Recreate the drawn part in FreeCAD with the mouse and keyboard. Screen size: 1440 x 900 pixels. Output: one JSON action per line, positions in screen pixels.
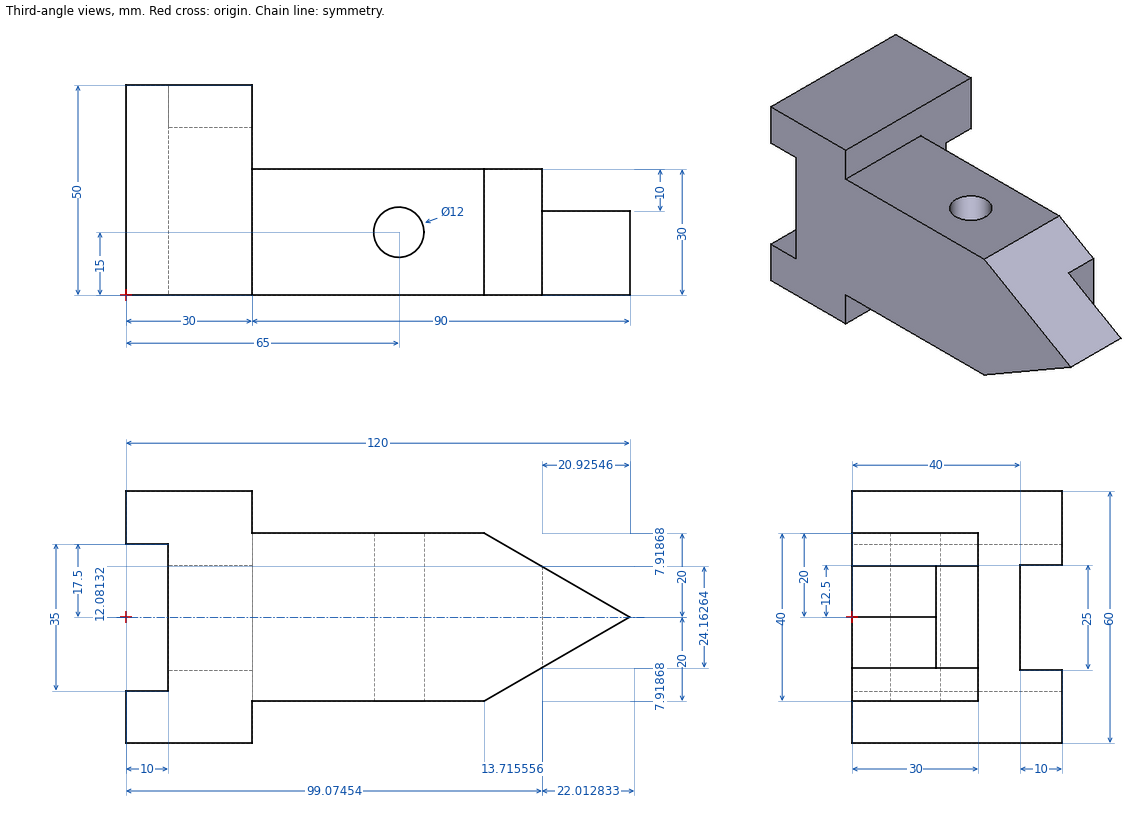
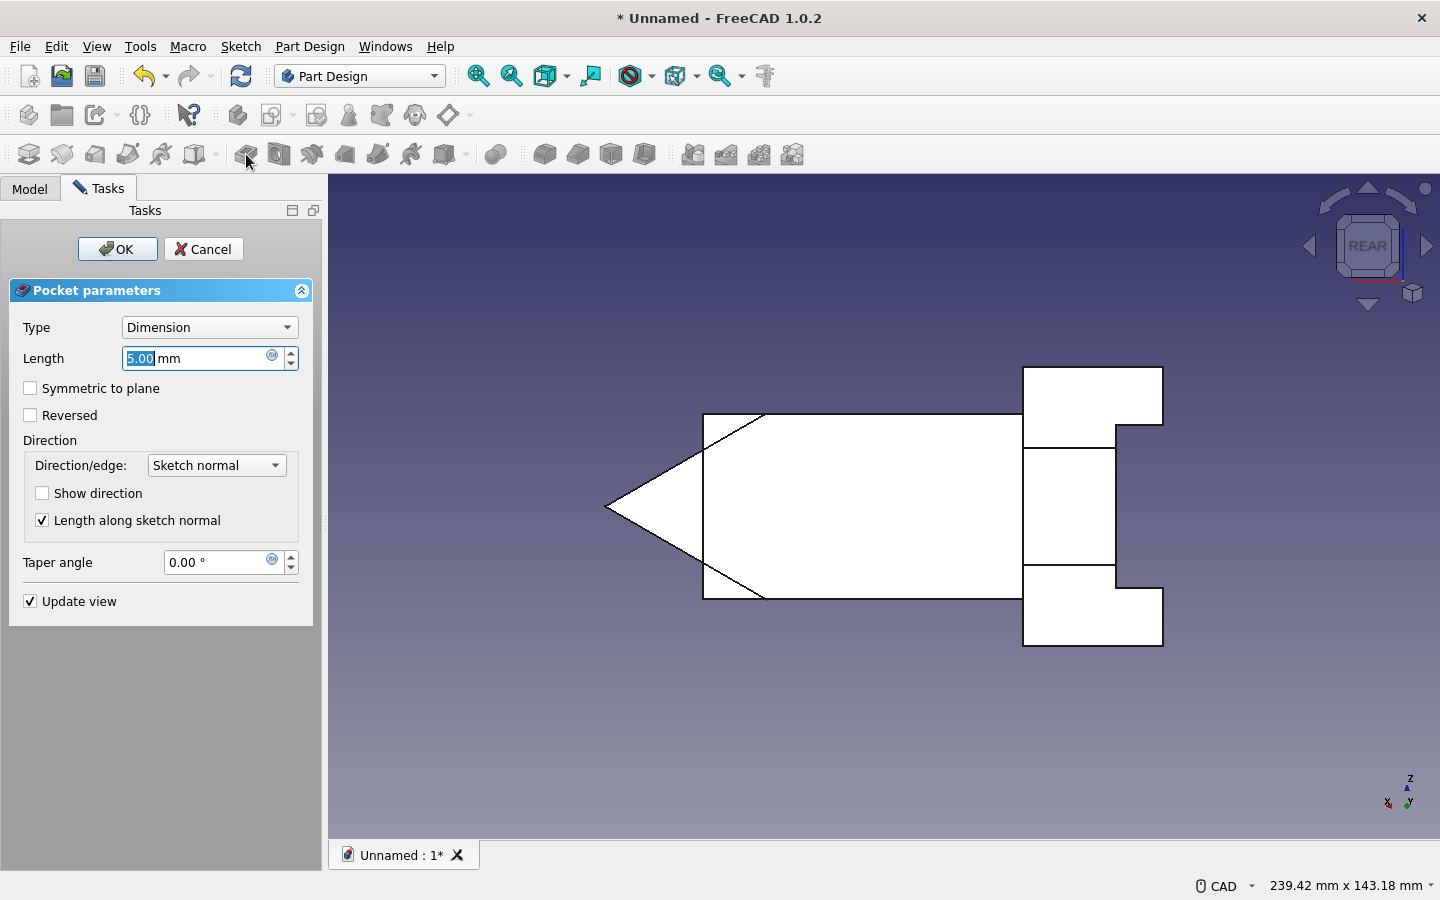
{"action": "type", "text": "30"}
{"action": "key", "text": "Tab"}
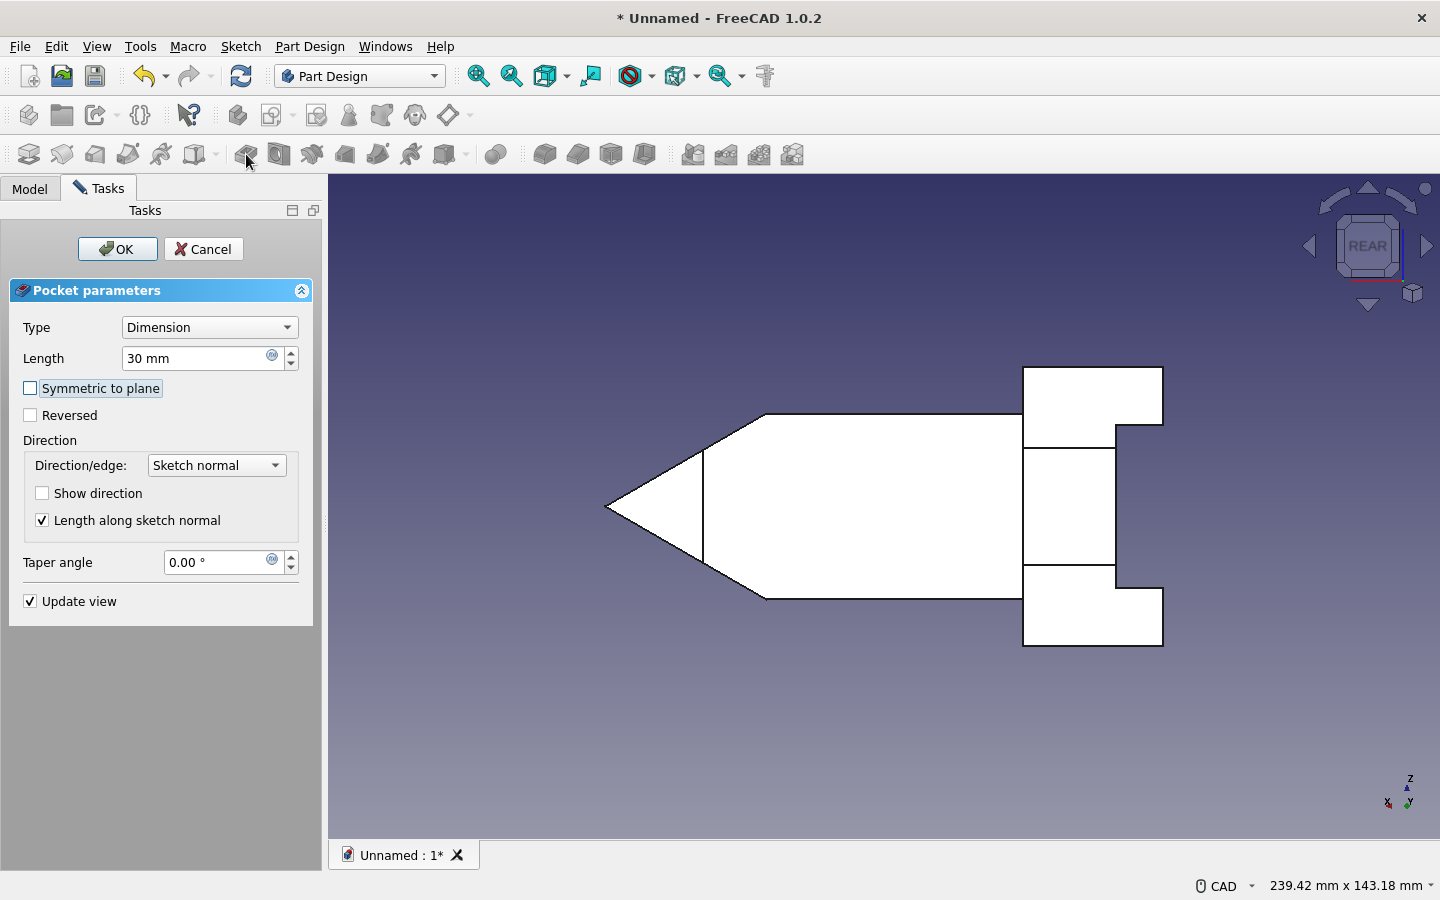
{"action": "left_click", "coordinate": [118, 249]}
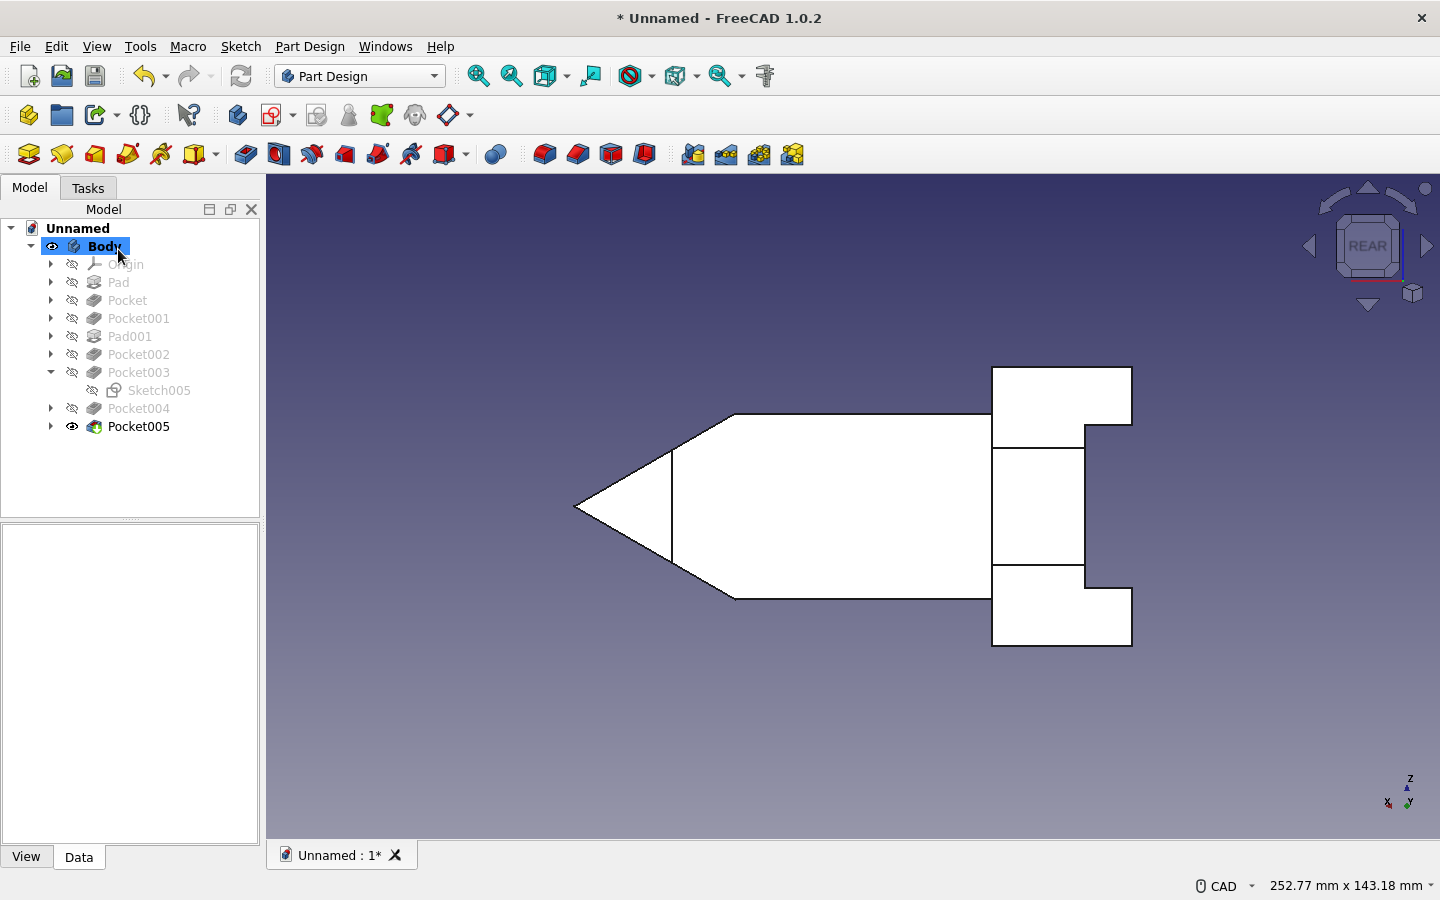
{"action": "key", "text": "0"}